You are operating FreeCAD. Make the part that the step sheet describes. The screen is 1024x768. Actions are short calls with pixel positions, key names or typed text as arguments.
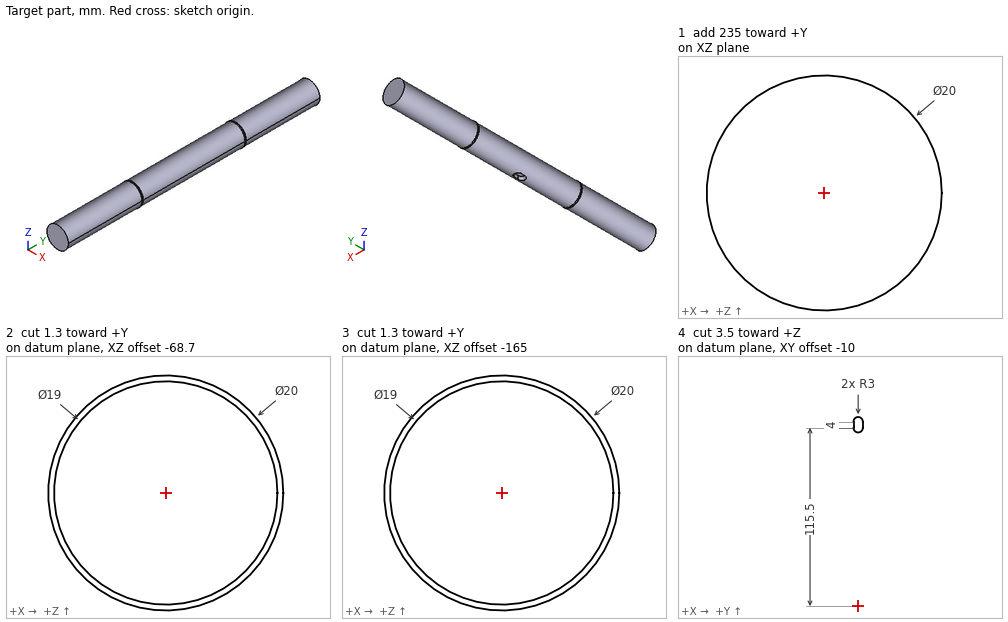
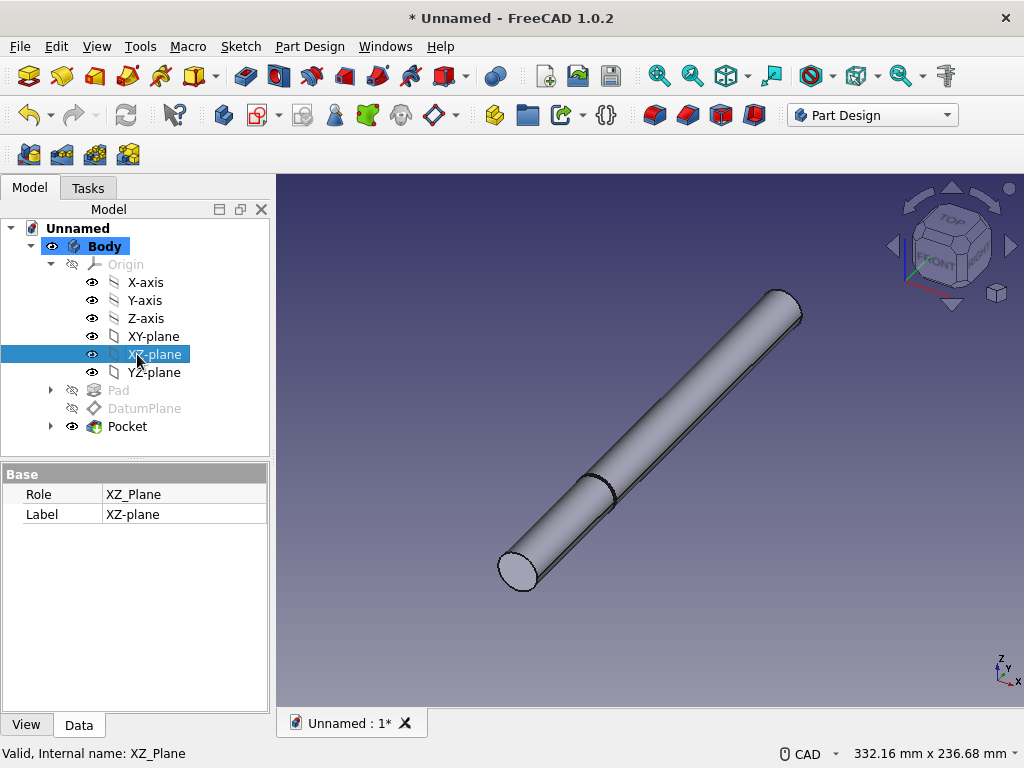
click(434, 116)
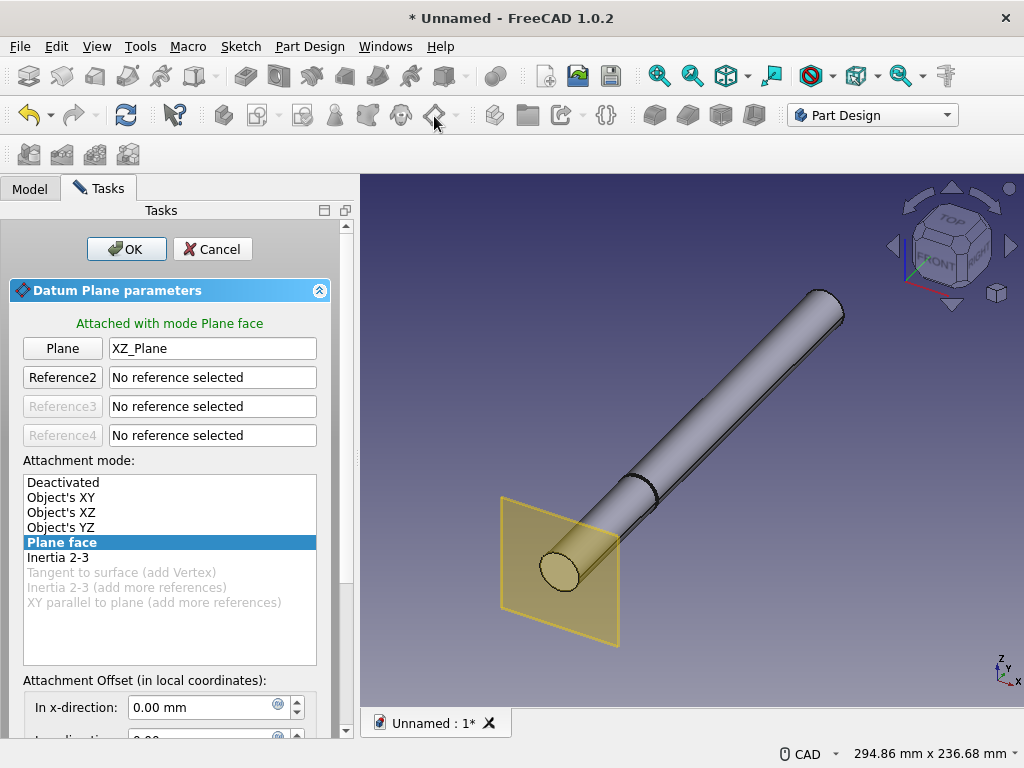
scroll(346, 479, down, 2)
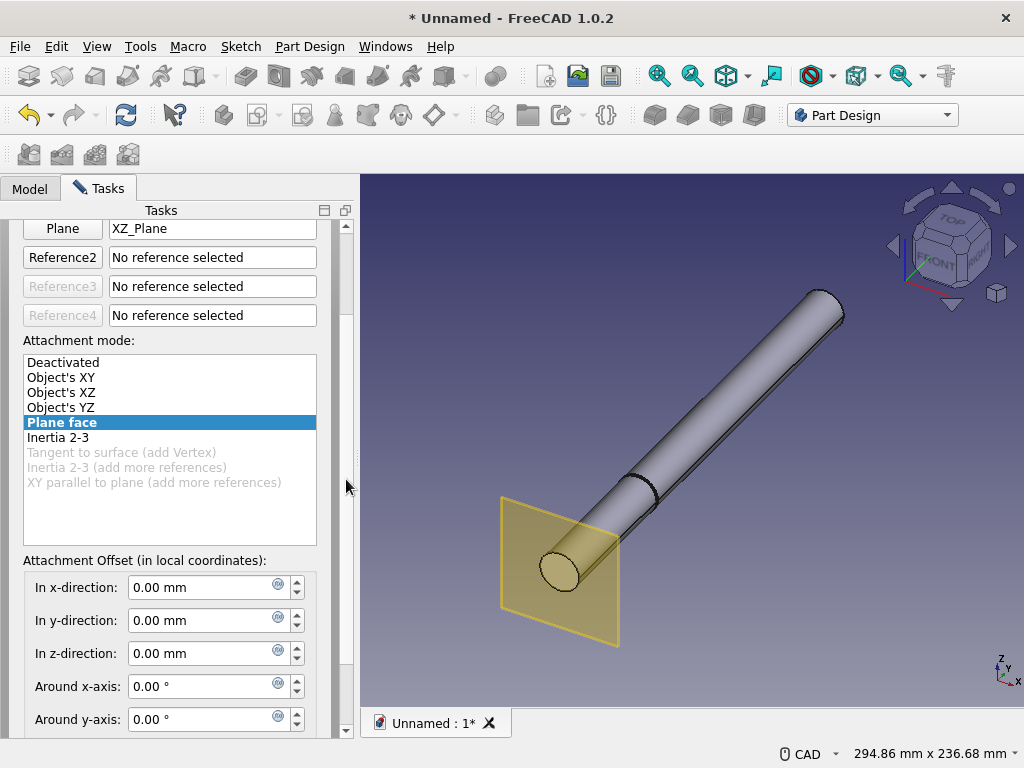
triple_click(210, 654)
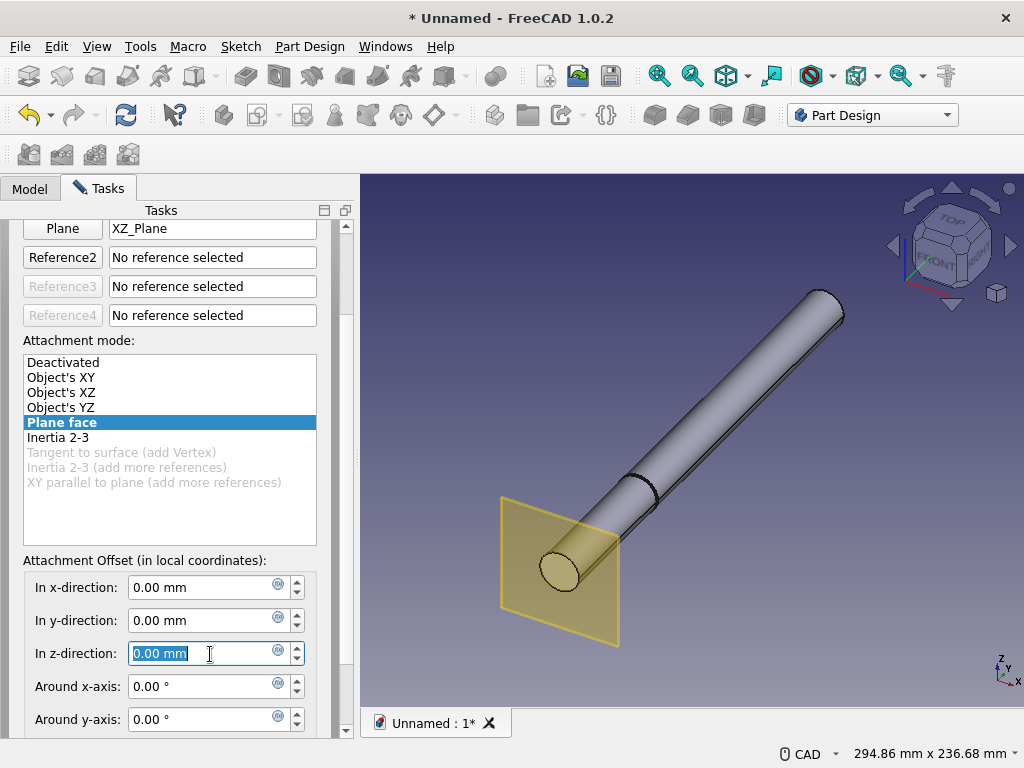
text(-165)
key(Tab)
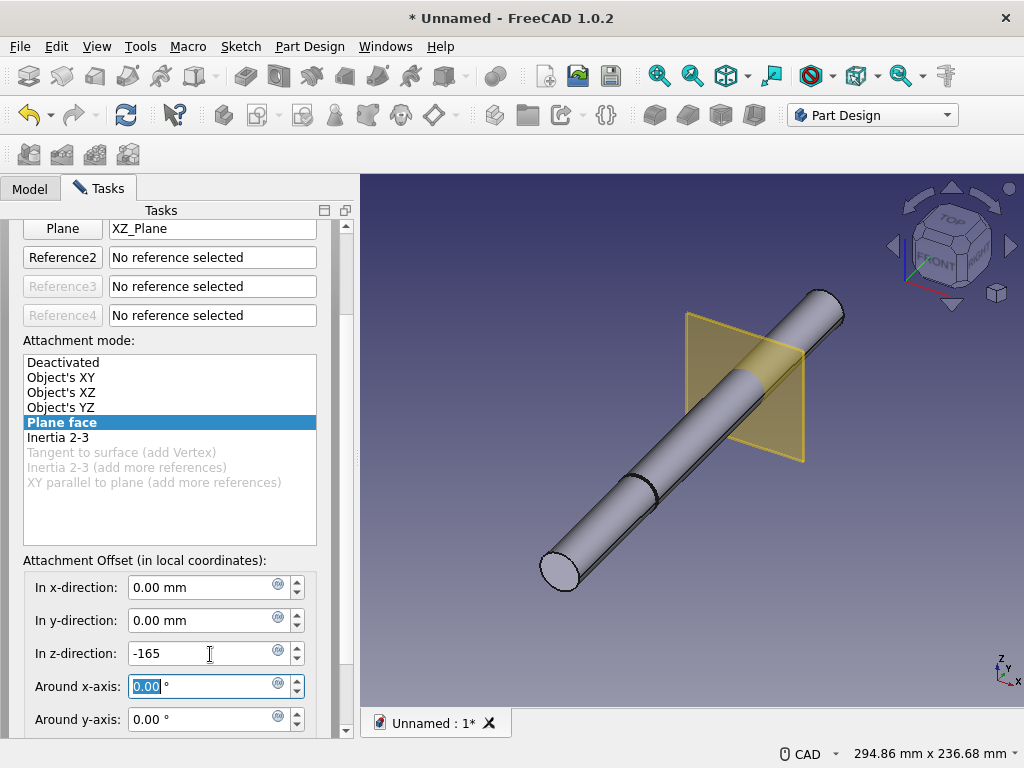
scroll(346, 479, up, 3)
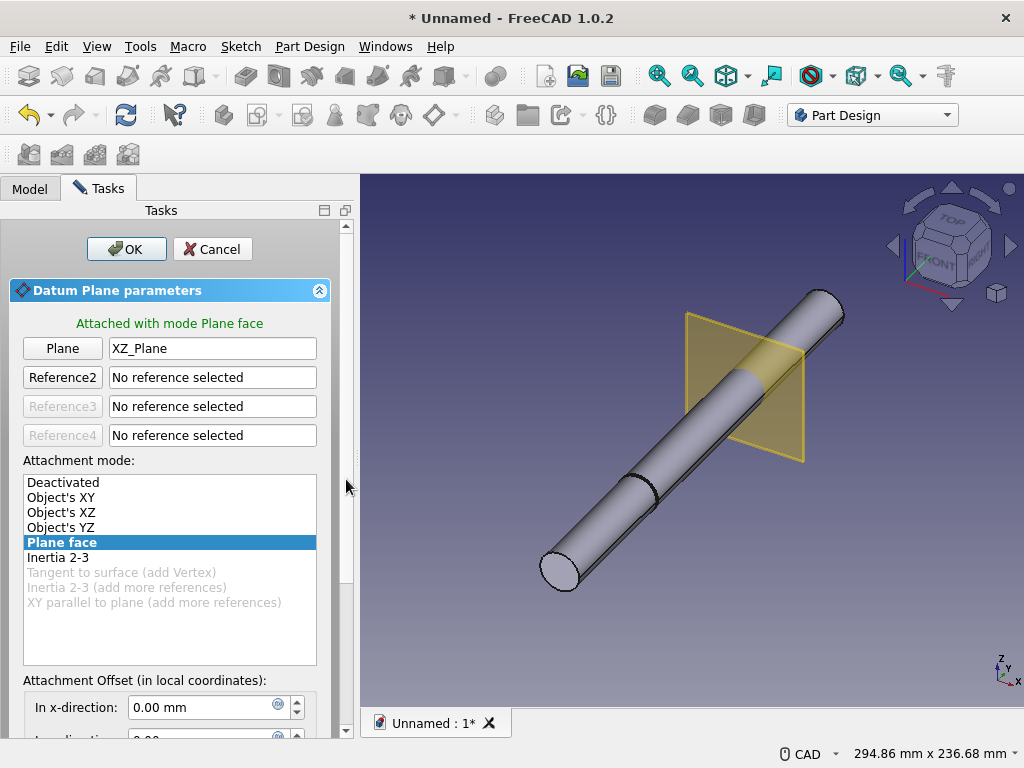
click(127, 249)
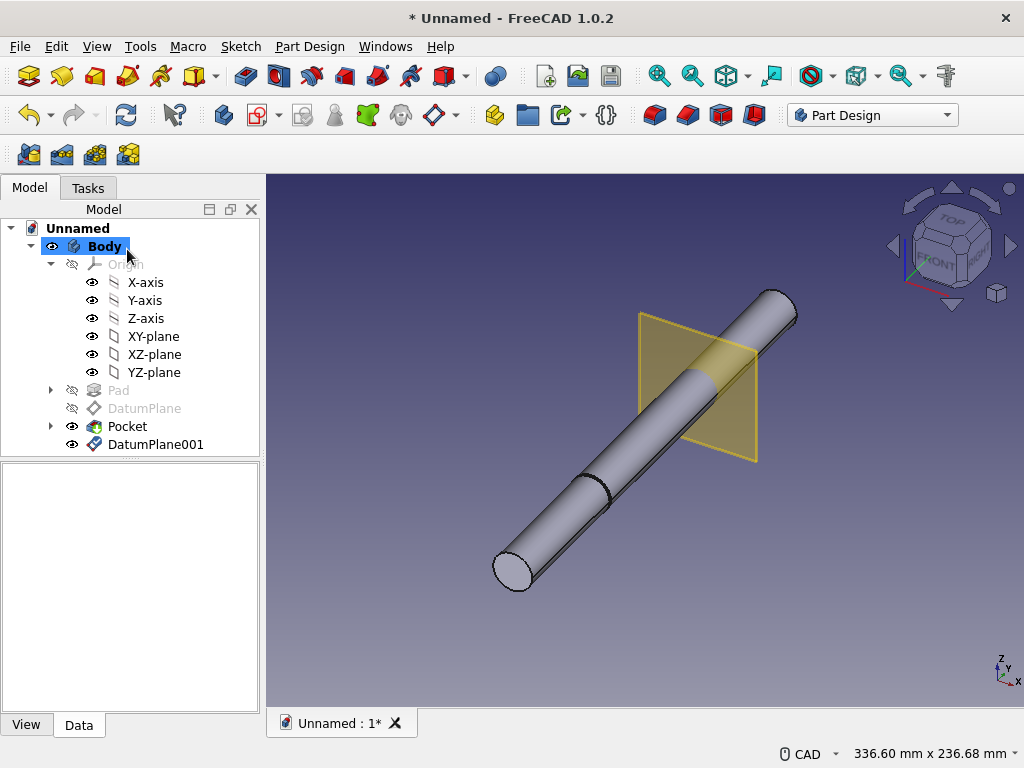
click(117, 444)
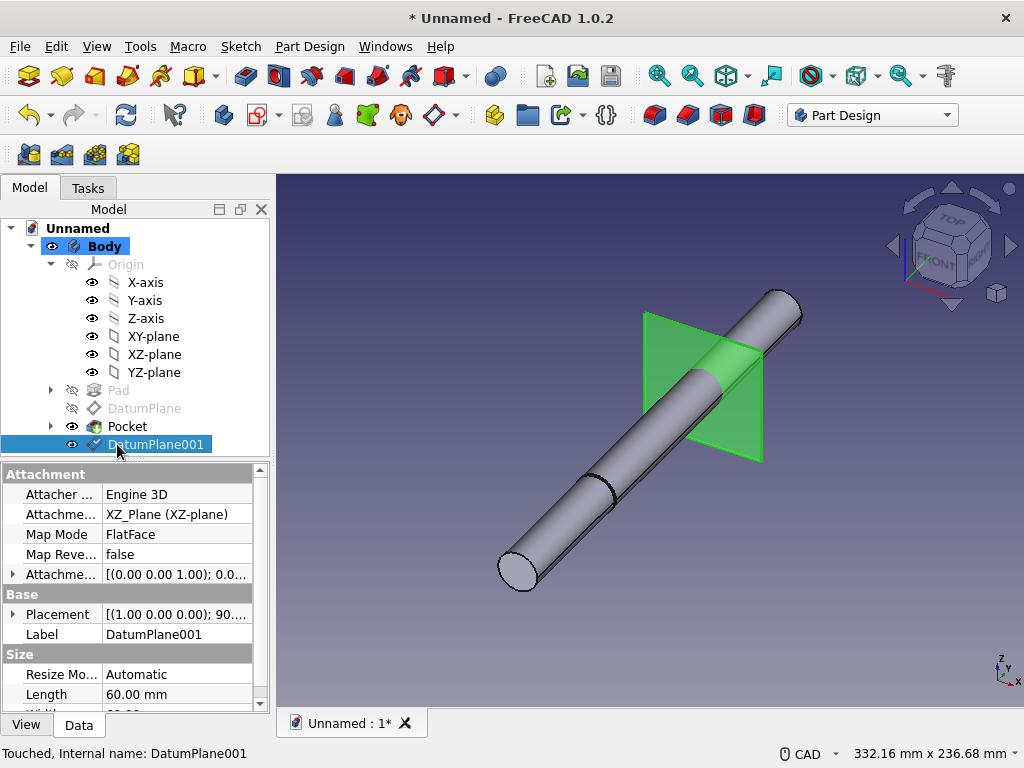
click(256, 116)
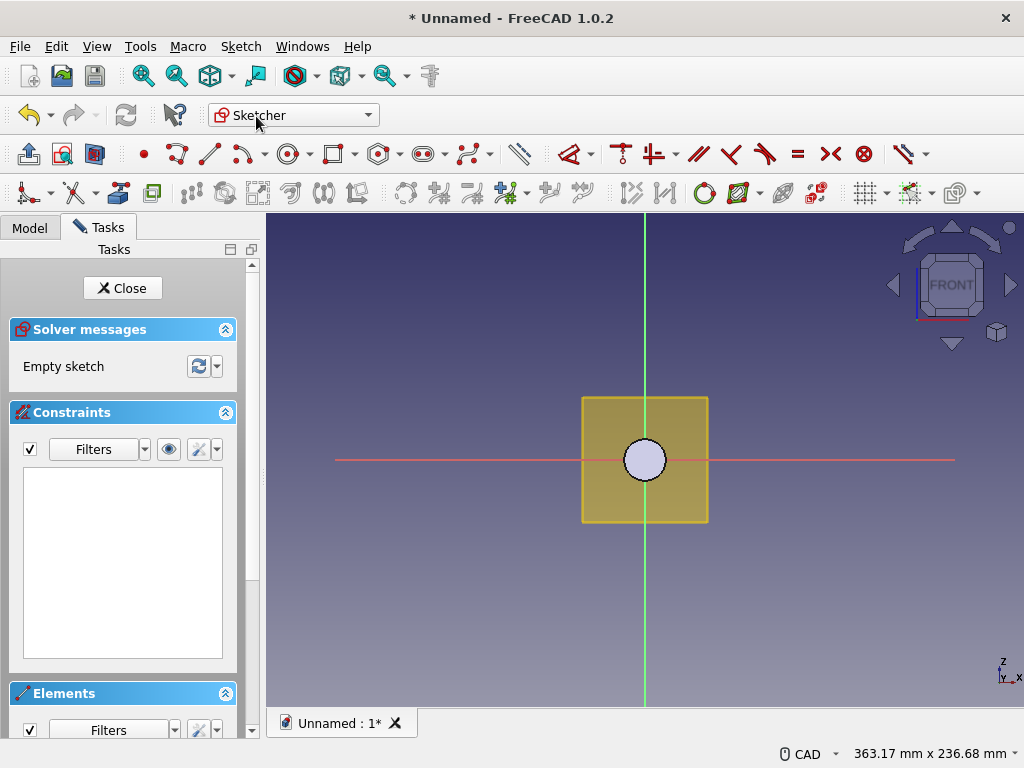
click(95, 154)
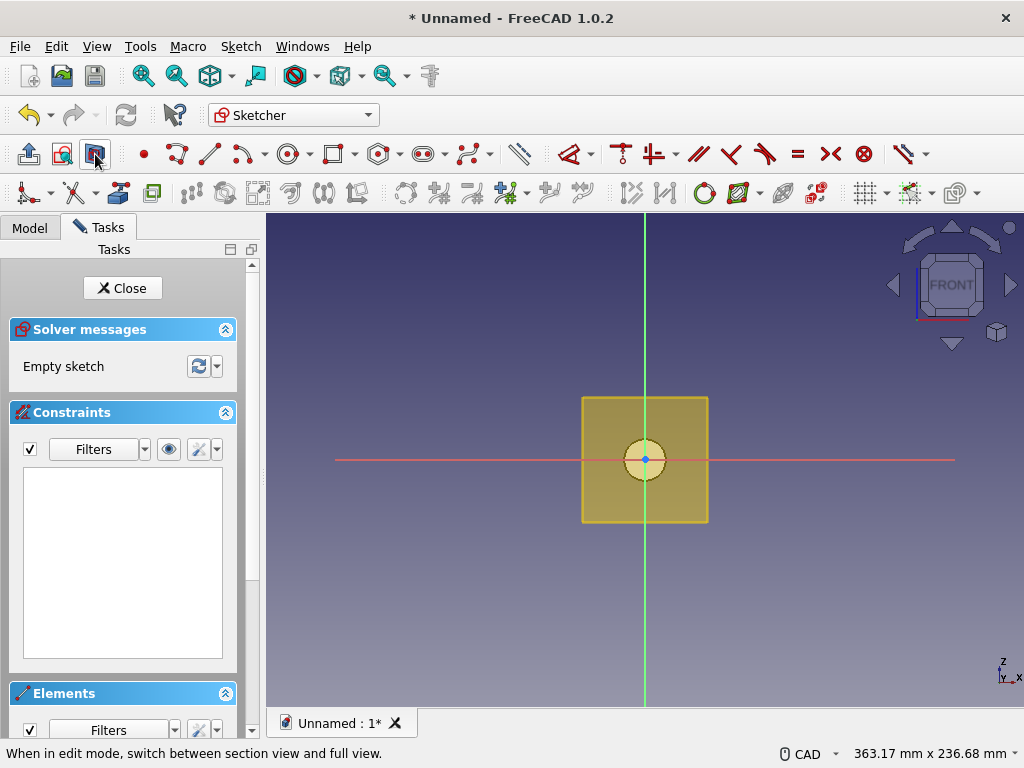
scroll(656, 460, up, 10)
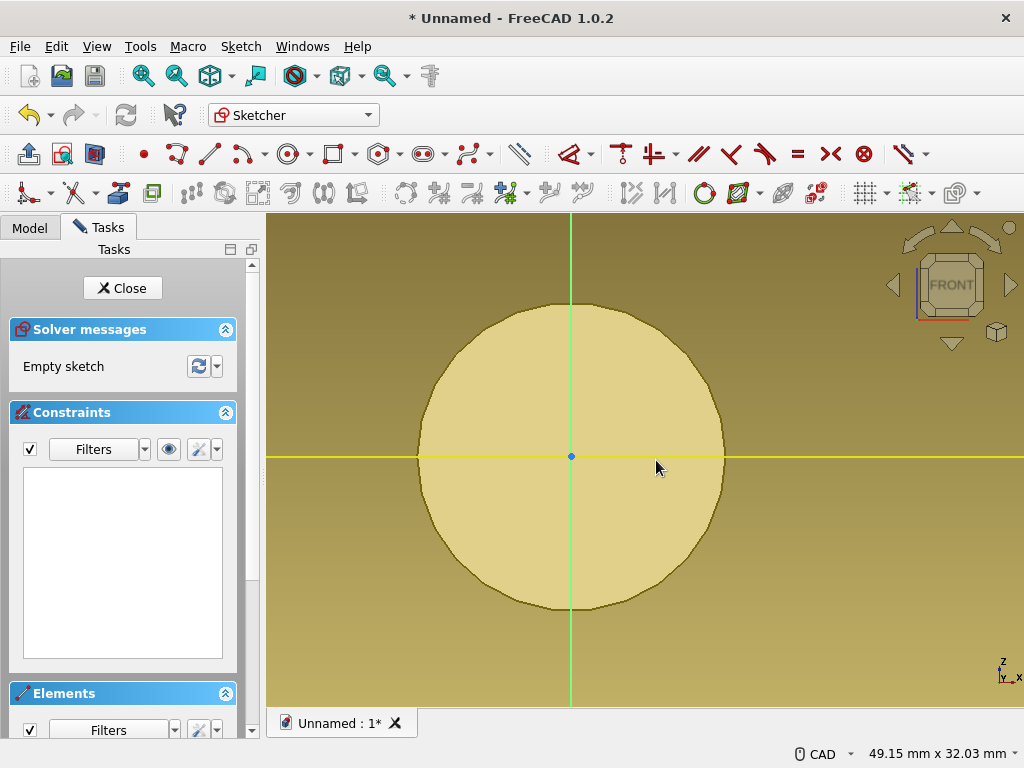
click(288, 154)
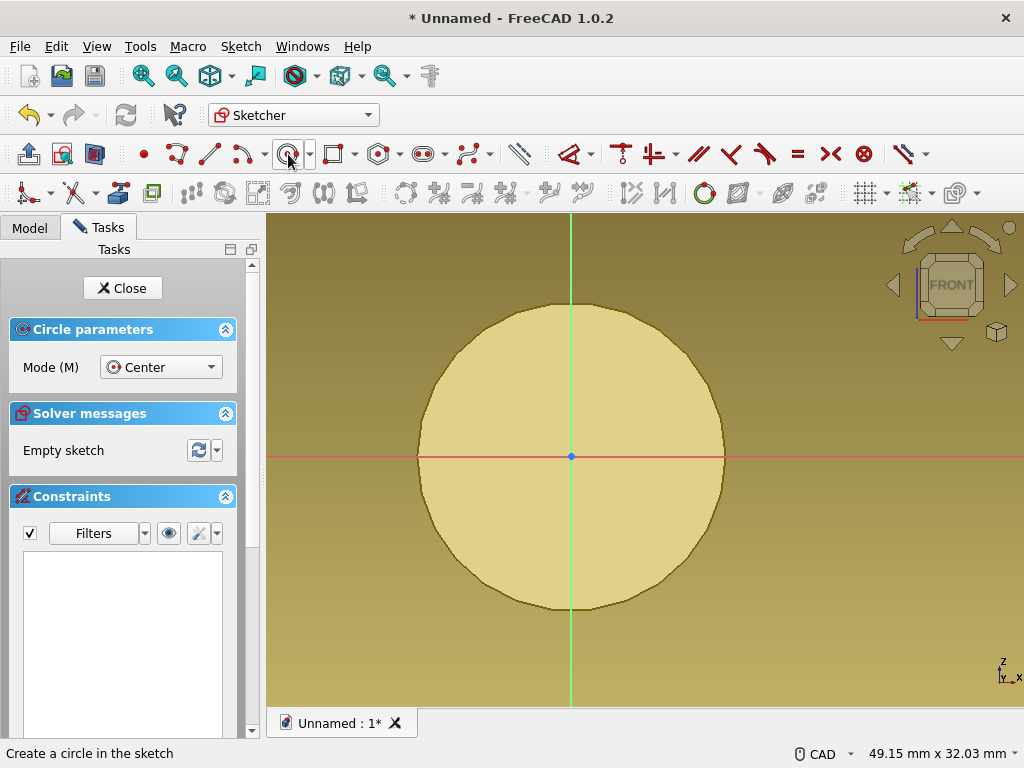
click(571, 457)
move(680, 348)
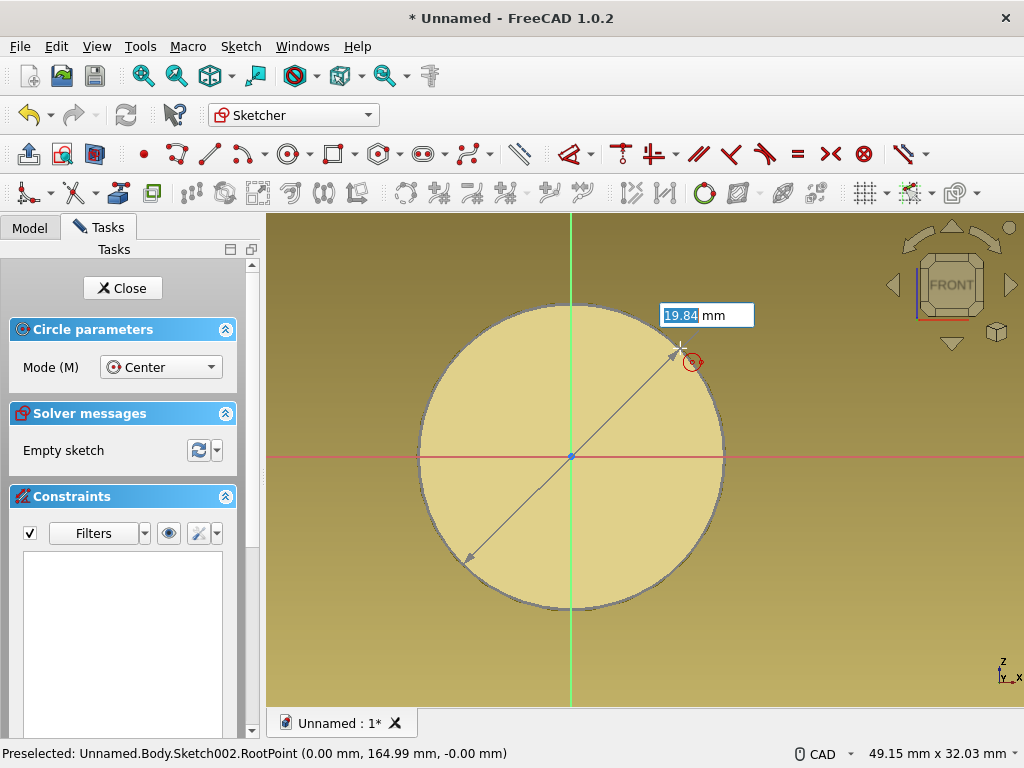
text(20)
key(Return)